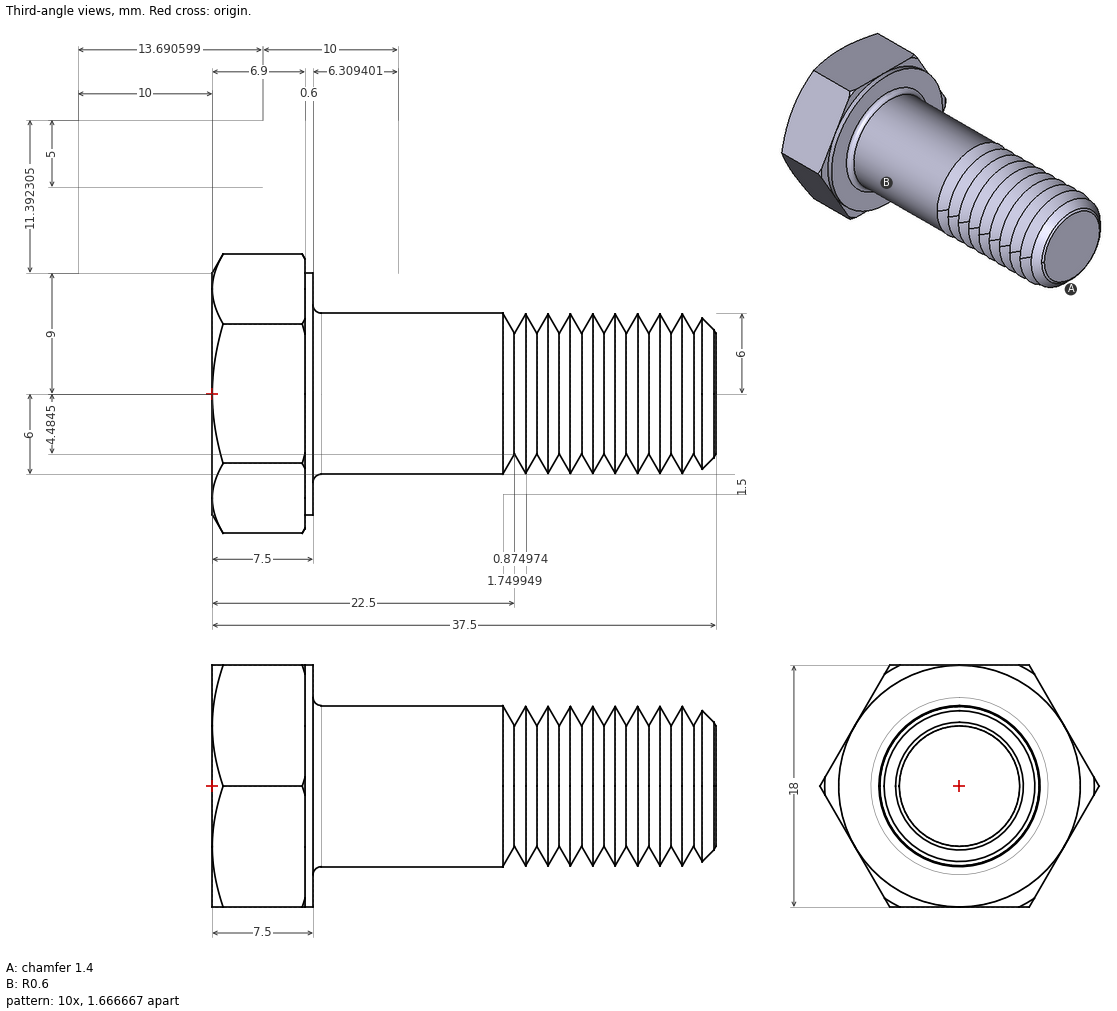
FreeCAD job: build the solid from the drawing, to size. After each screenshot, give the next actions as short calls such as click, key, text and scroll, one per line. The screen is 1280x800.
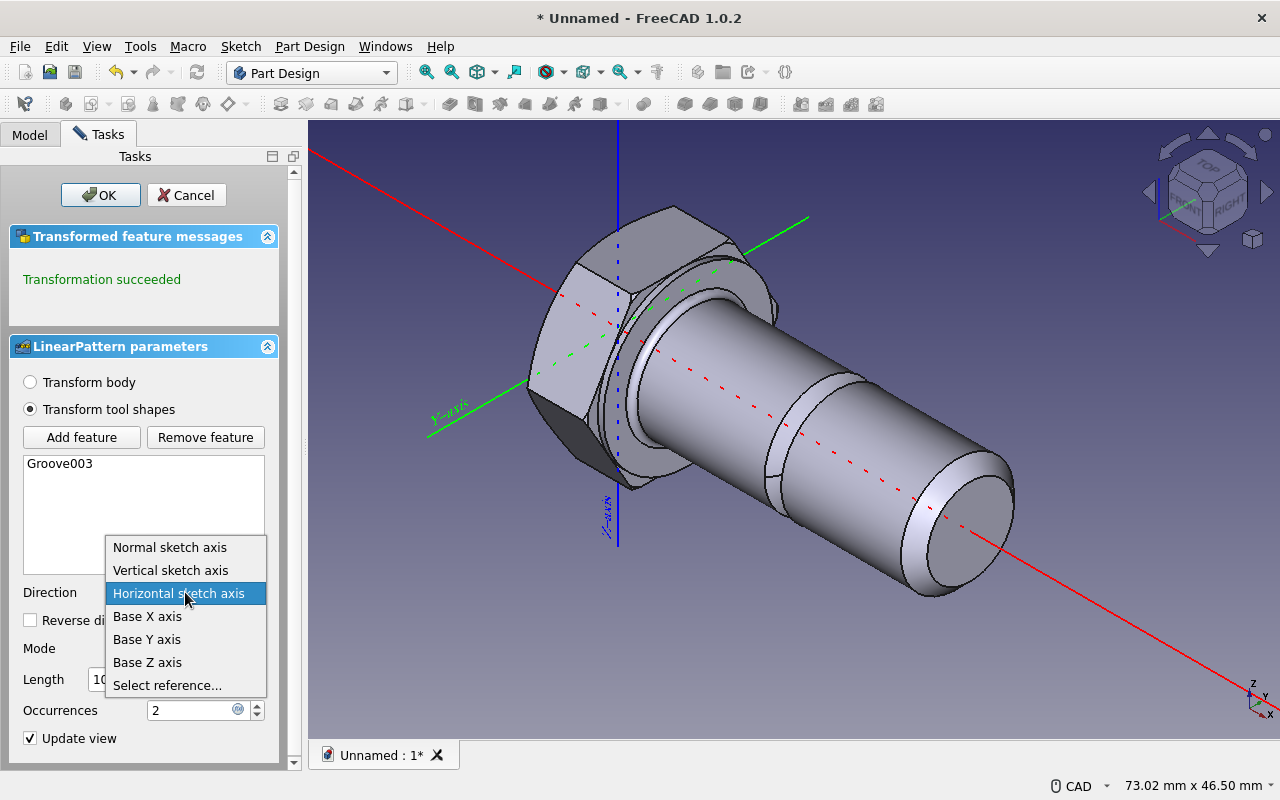
click(184, 616)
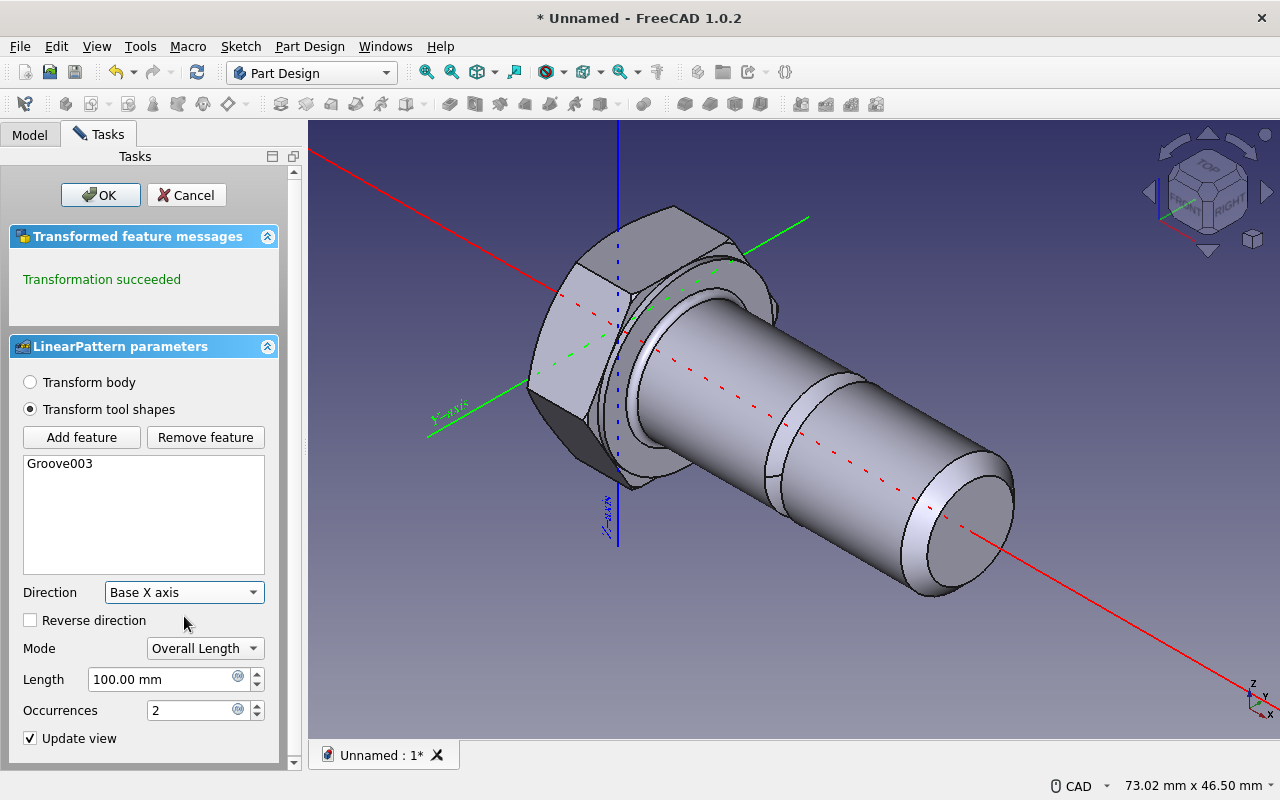
click(206, 648)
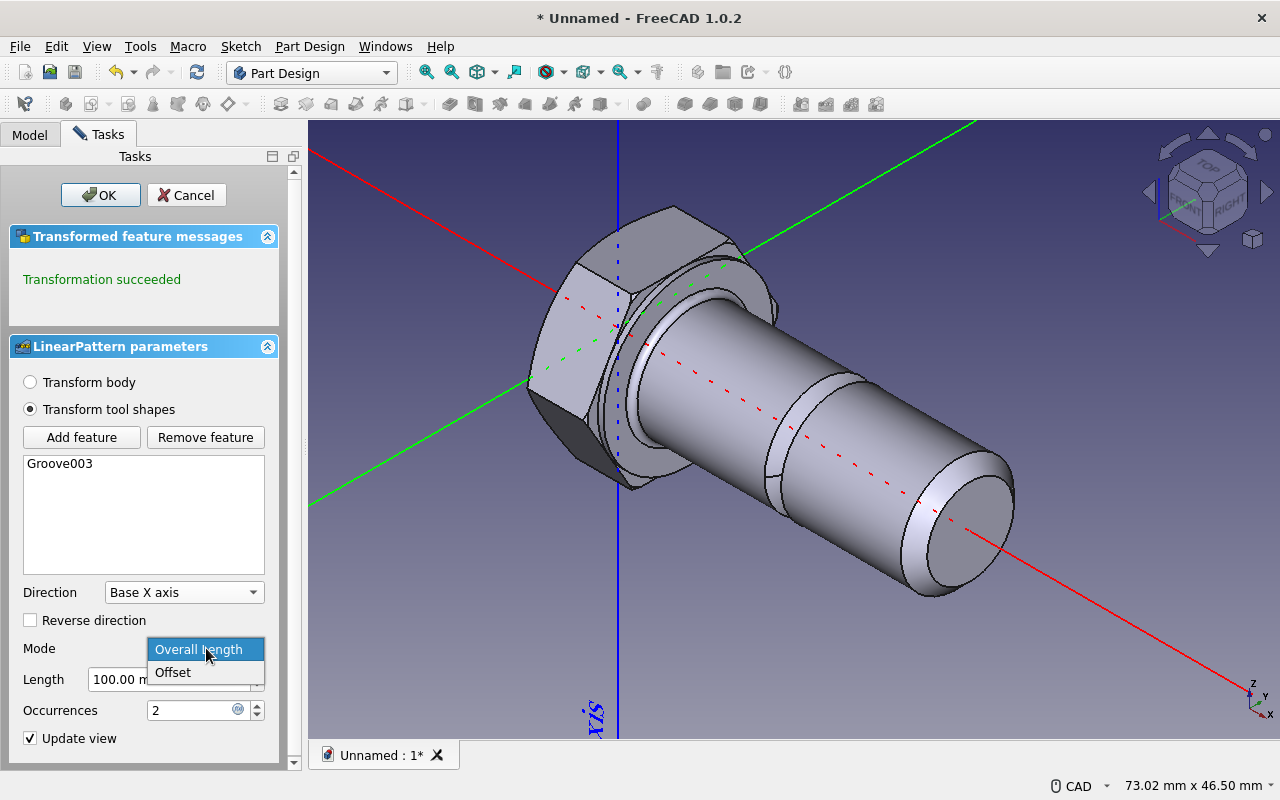
click(204, 672)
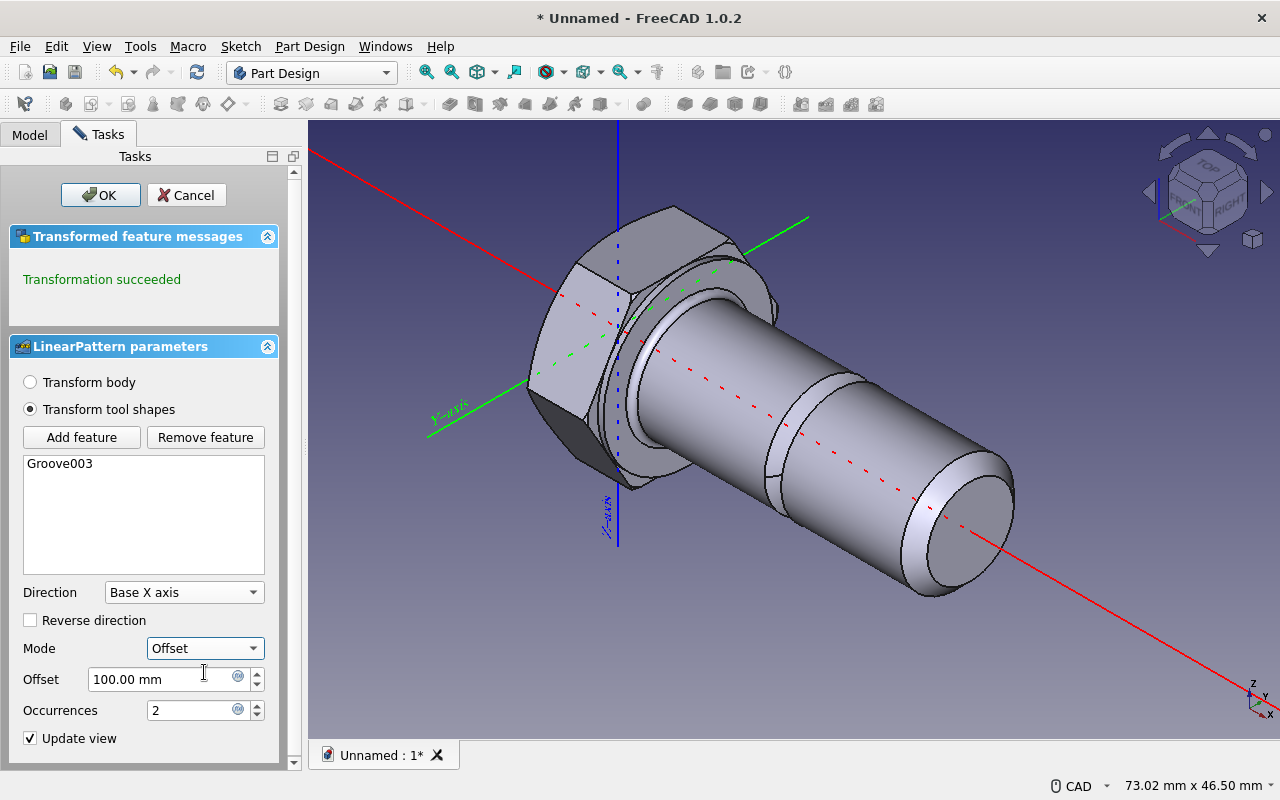
triple_click(170, 680)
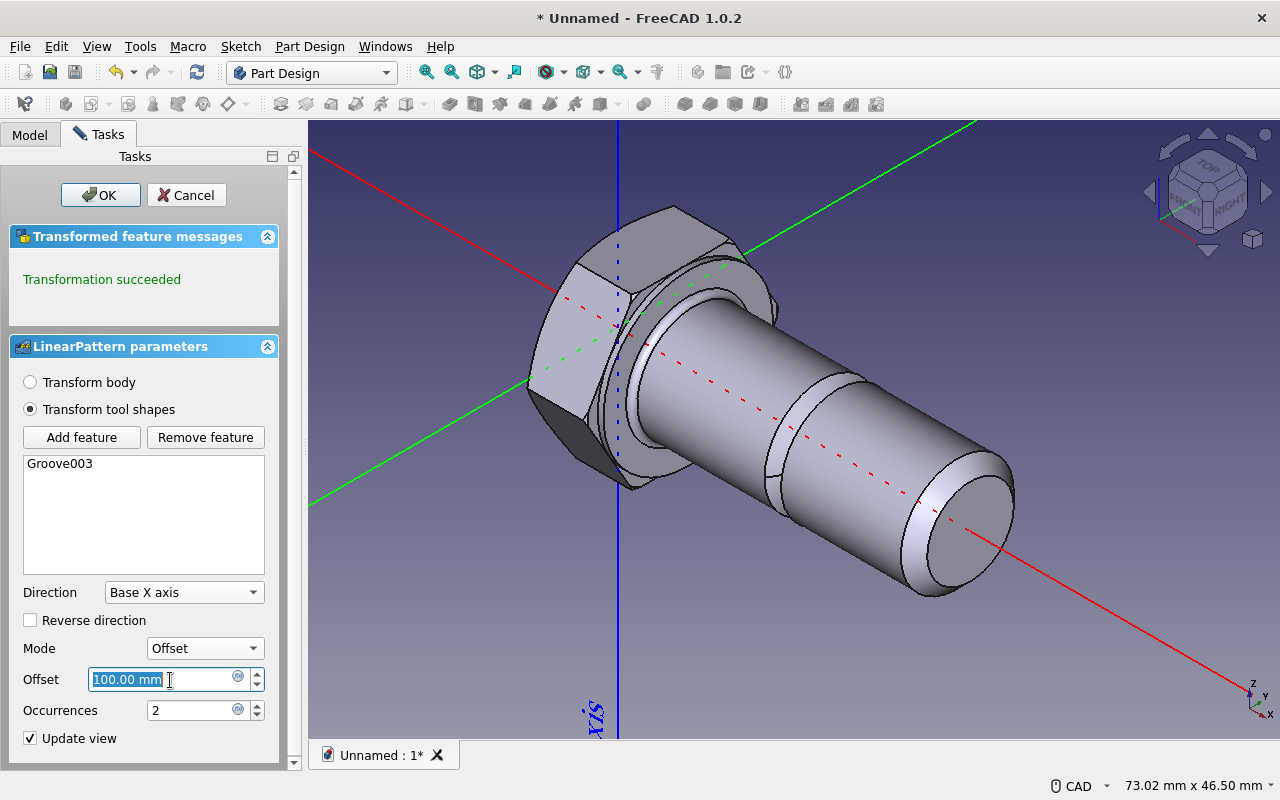
text(1.666667)
key(Tab)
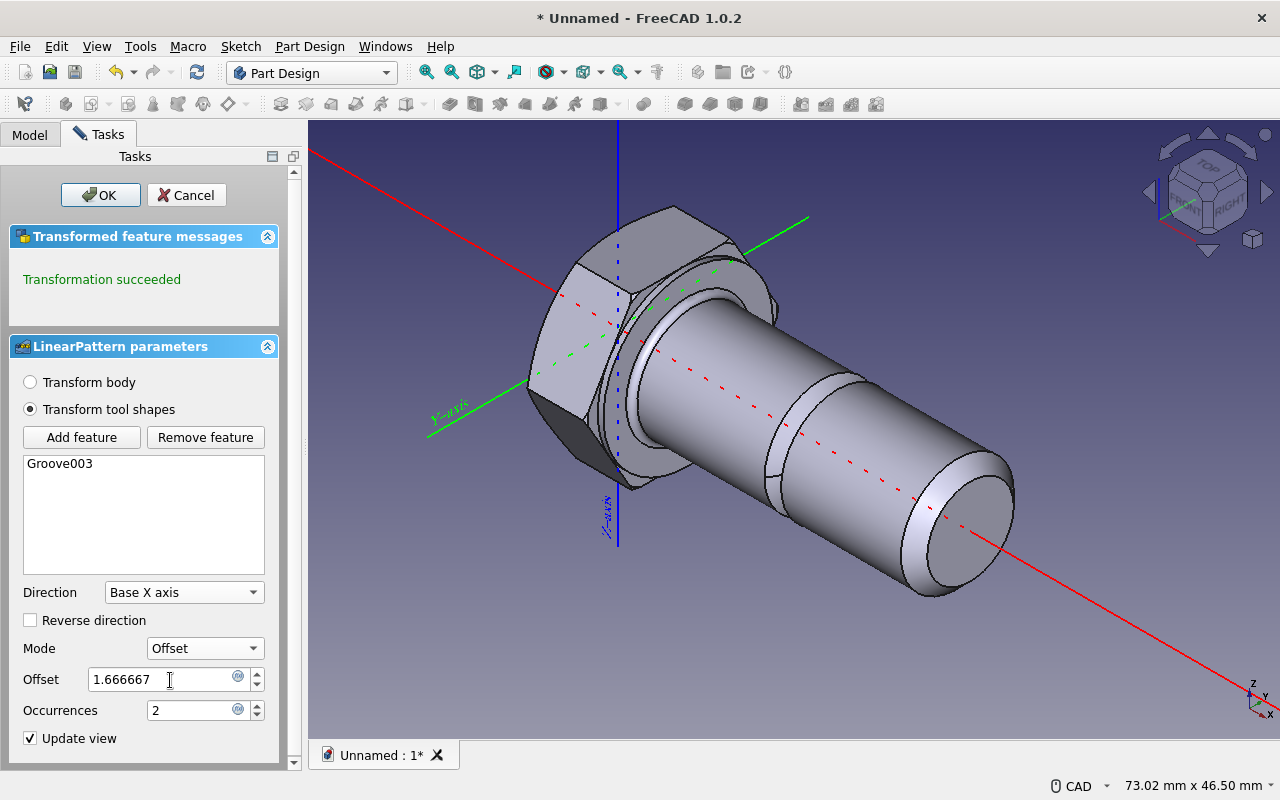
triple_click(199, 710)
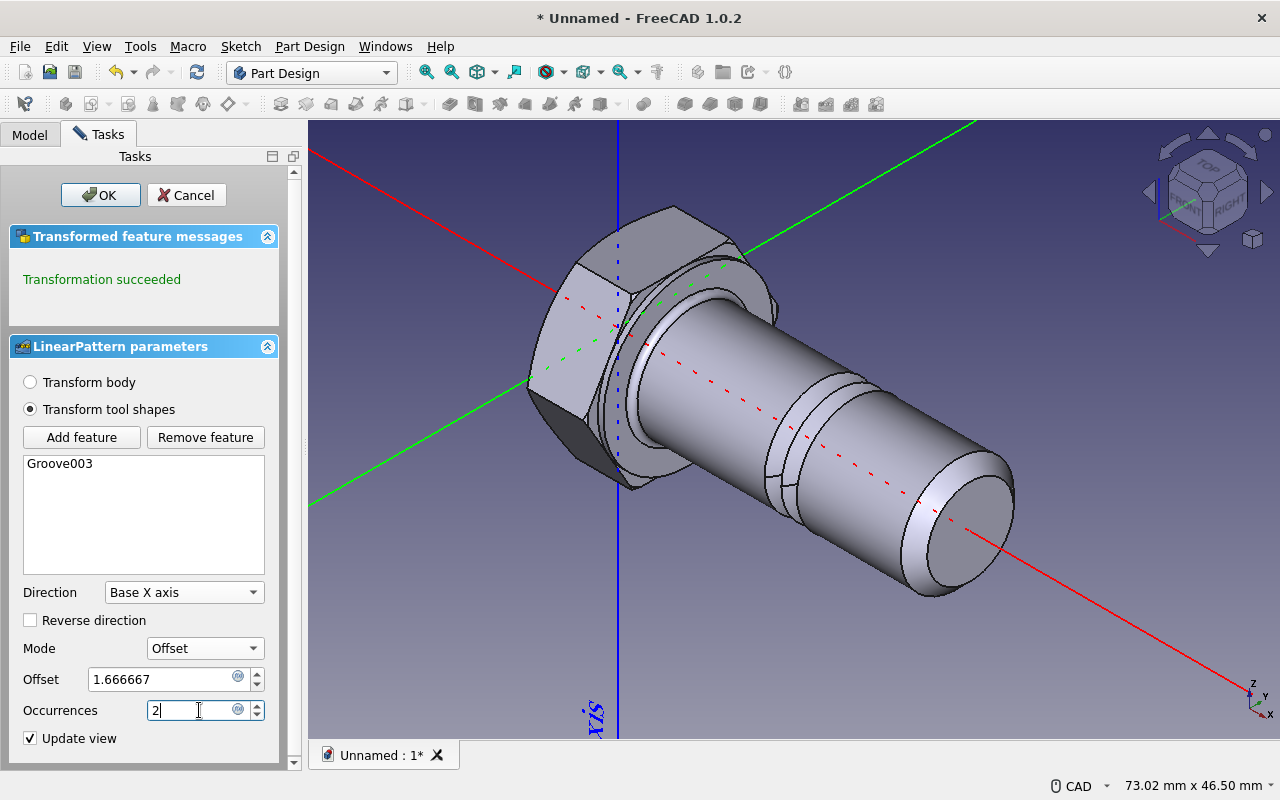
text(10)
key(Tab)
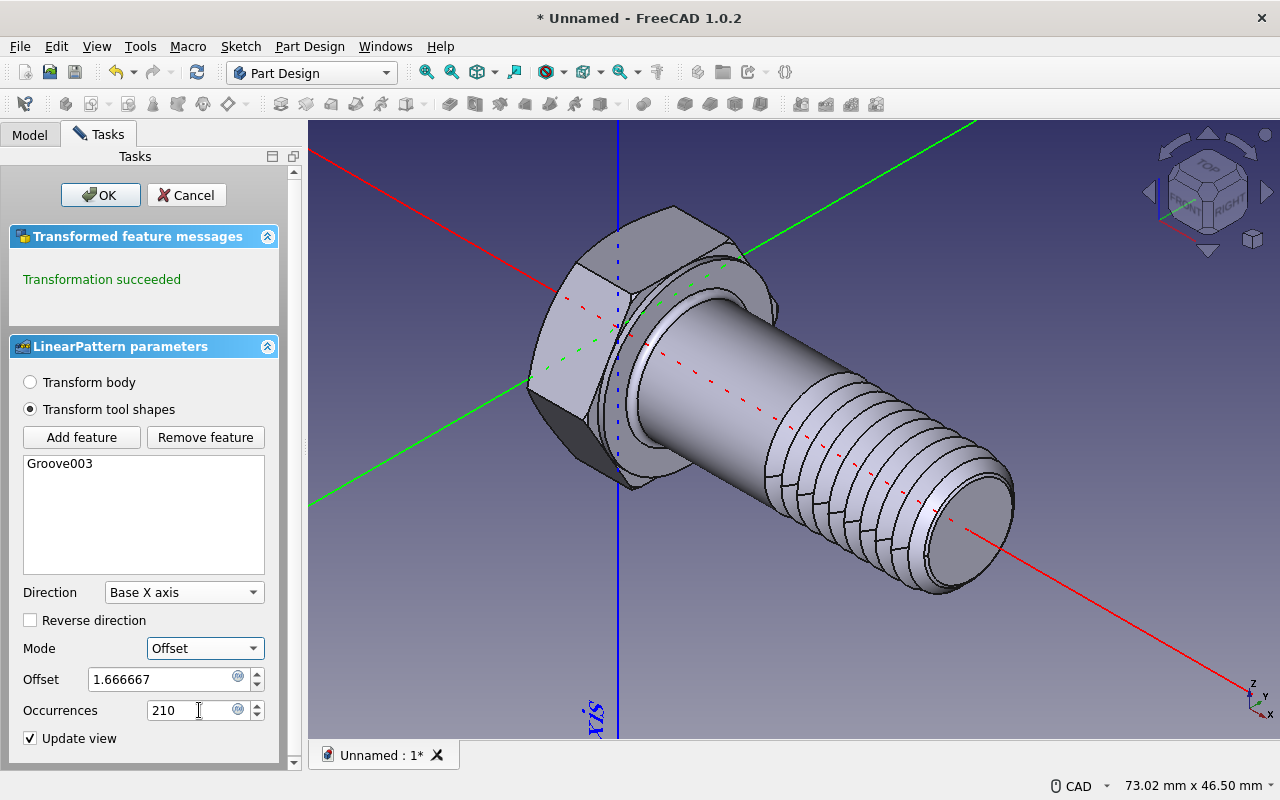
click(101, 195)